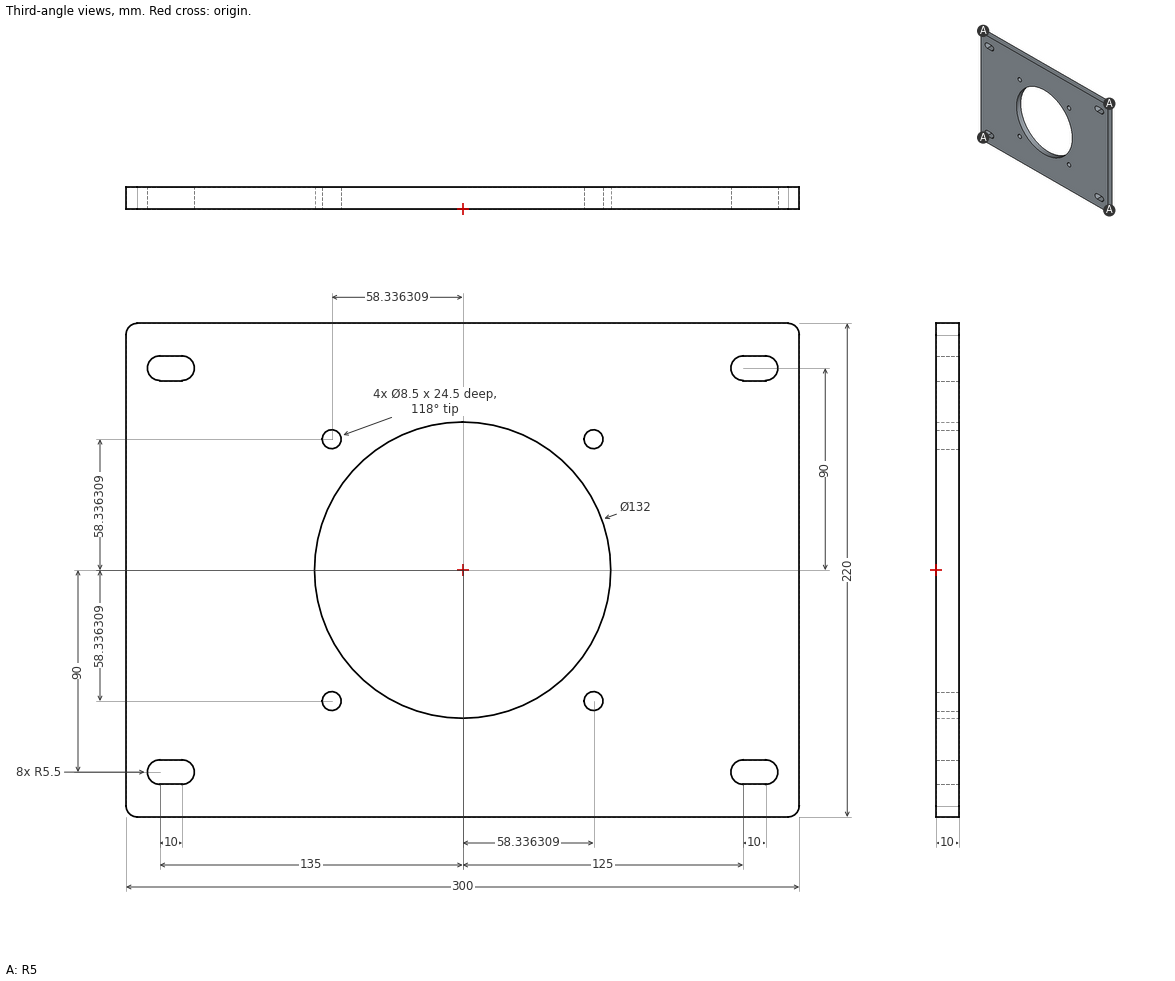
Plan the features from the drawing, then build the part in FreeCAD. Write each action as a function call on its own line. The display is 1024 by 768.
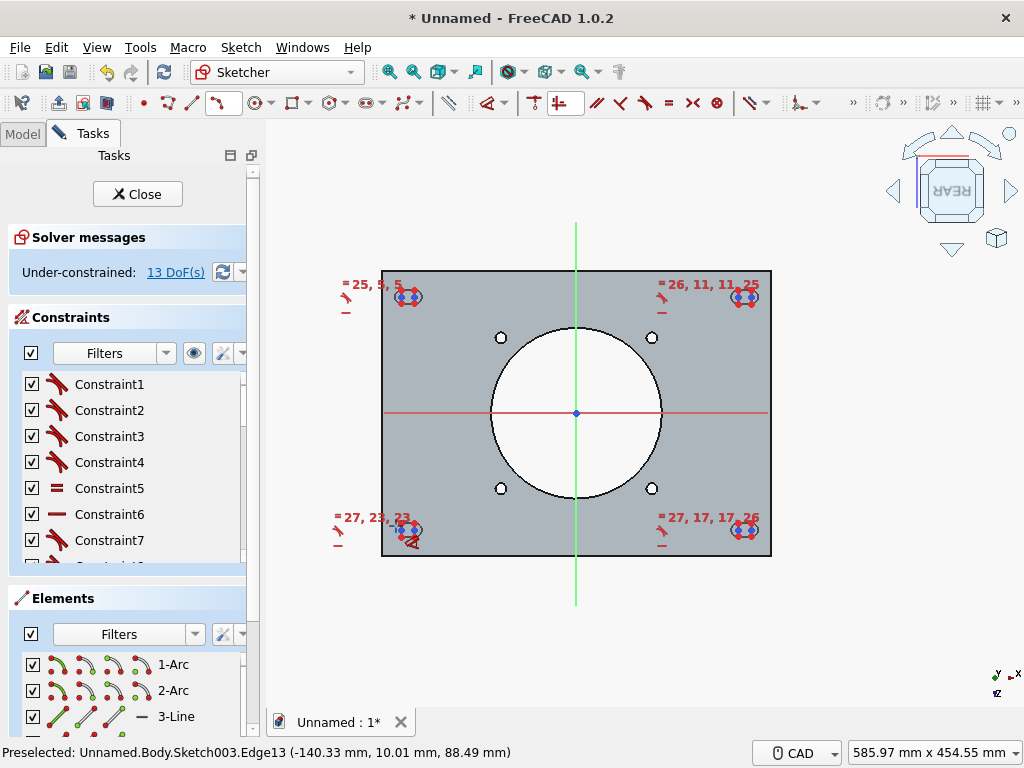
scroll(396, 293, up, 9)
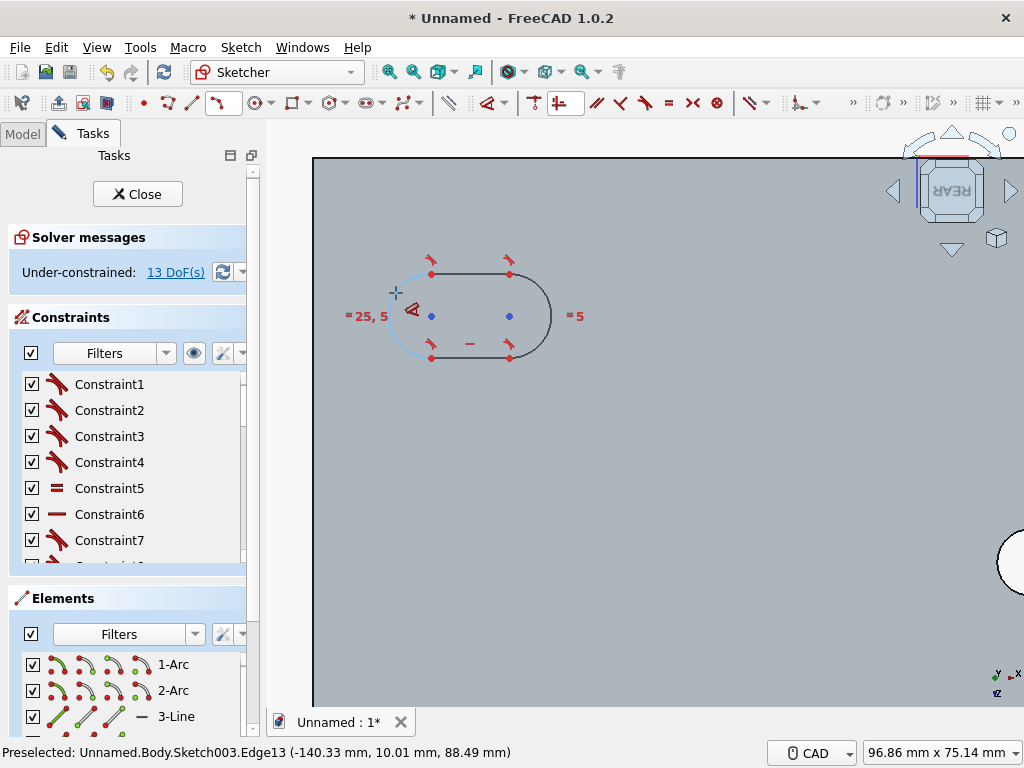
click(397, 291)
click(371, 272)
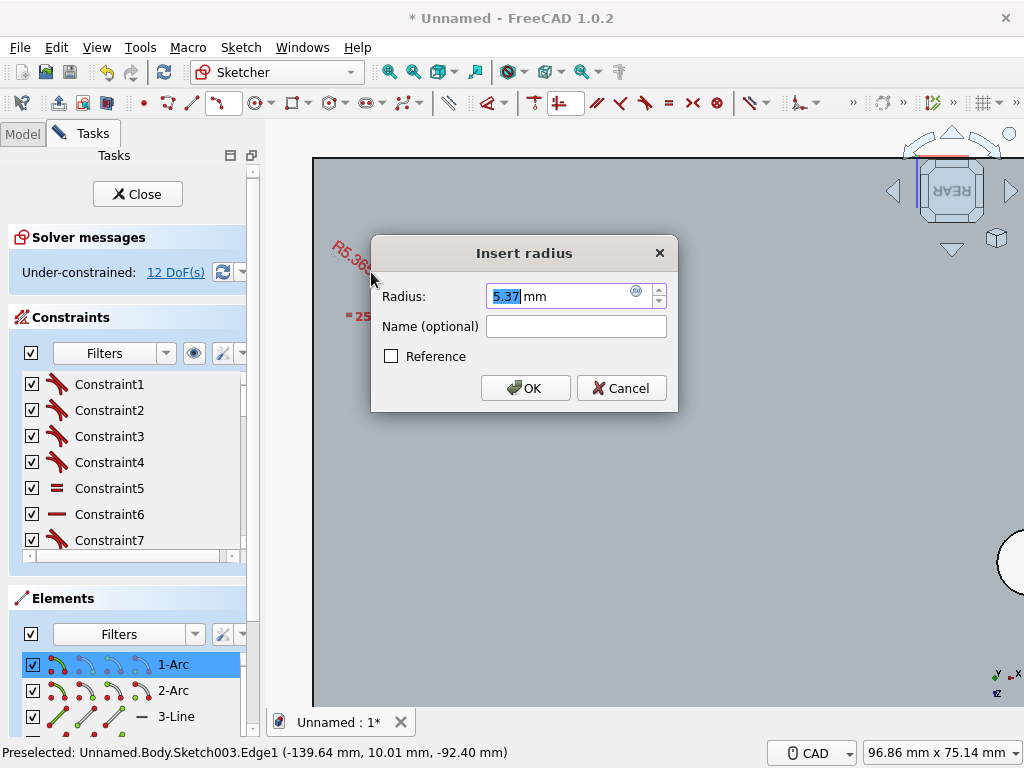
text(5.5)
key(Return)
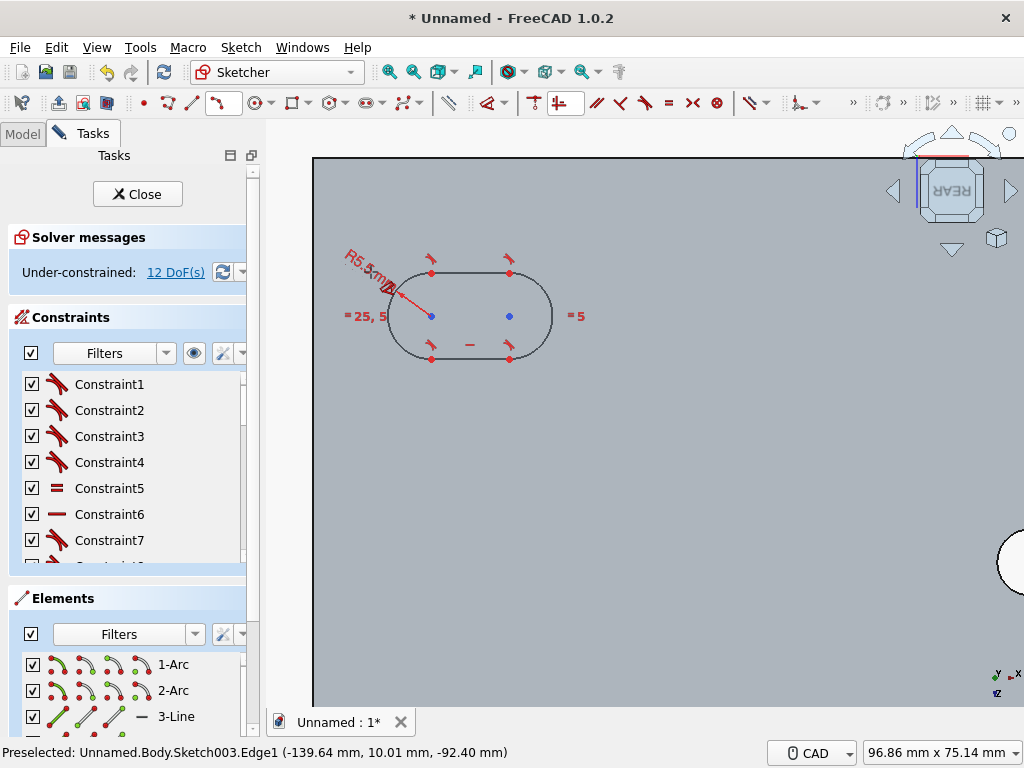
click(455, 273)
click(470, 239)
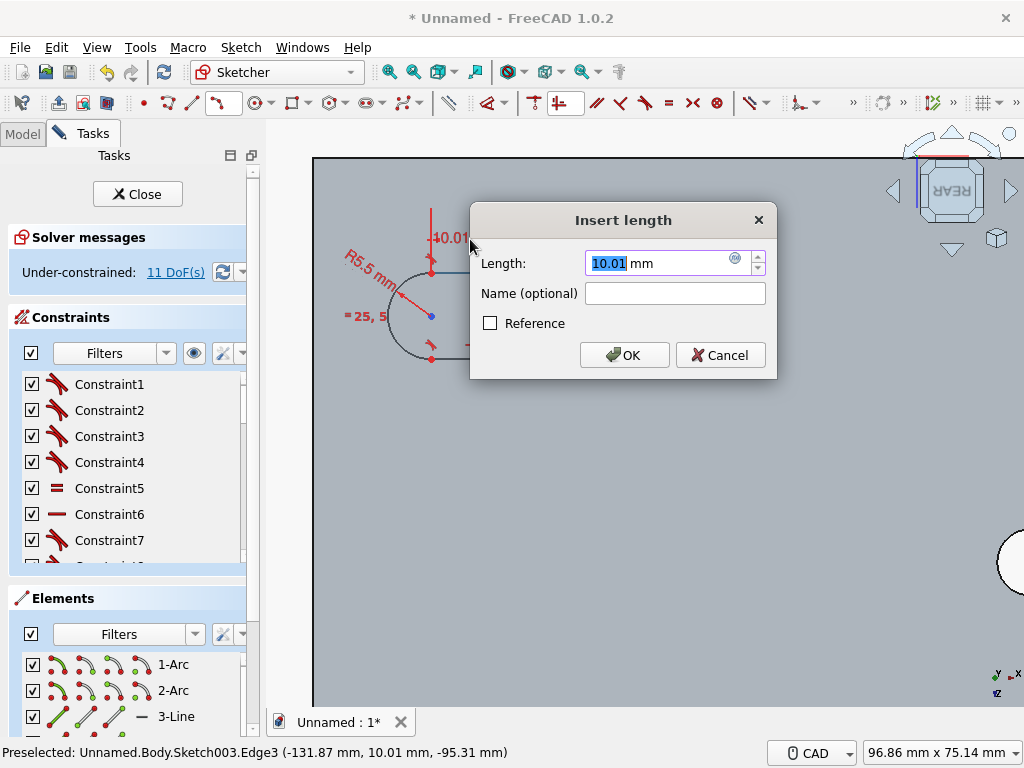
text(10)
key(Return)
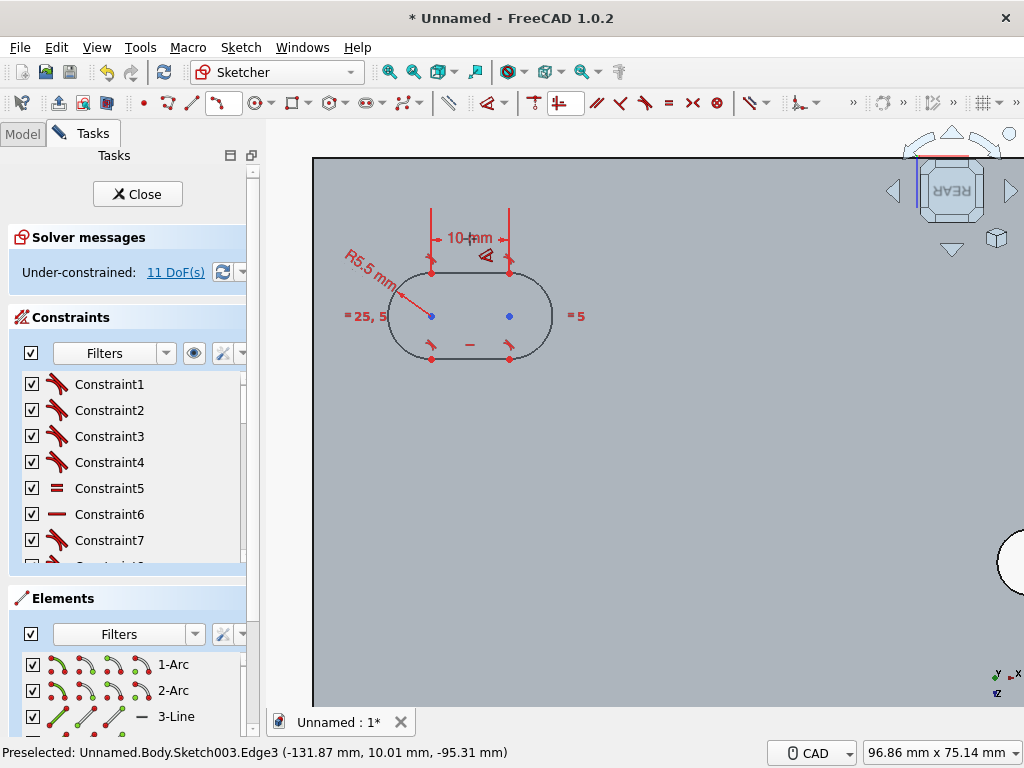
scroll(396, 293, down, 9)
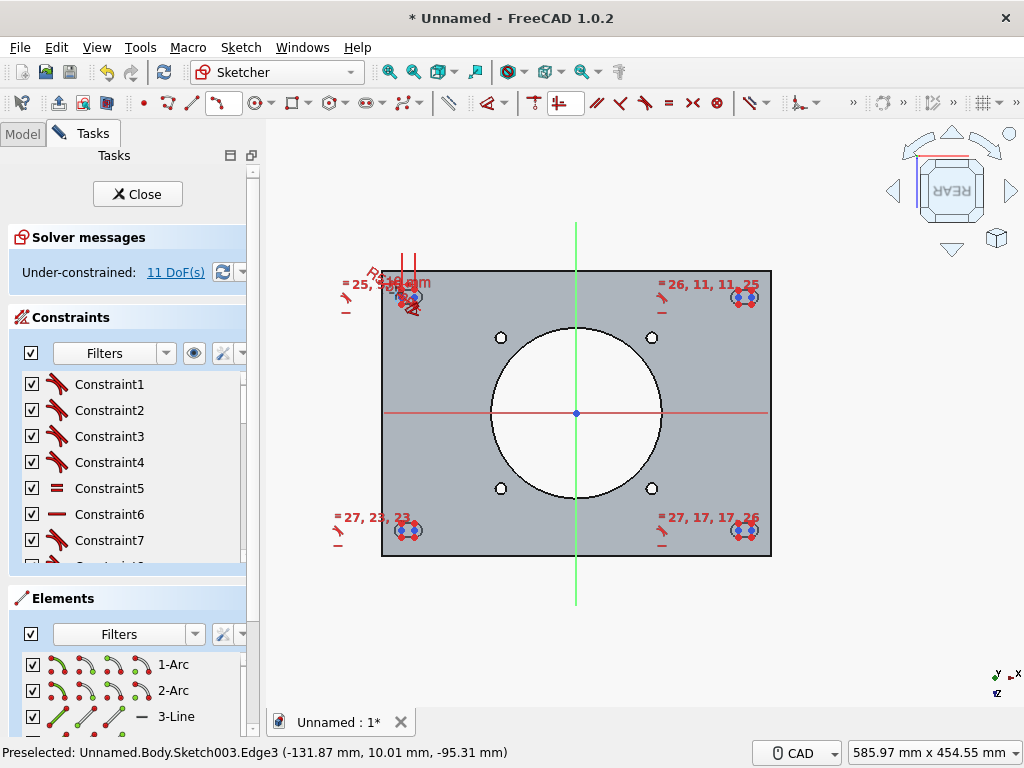
scroll(742, 290, up, 7)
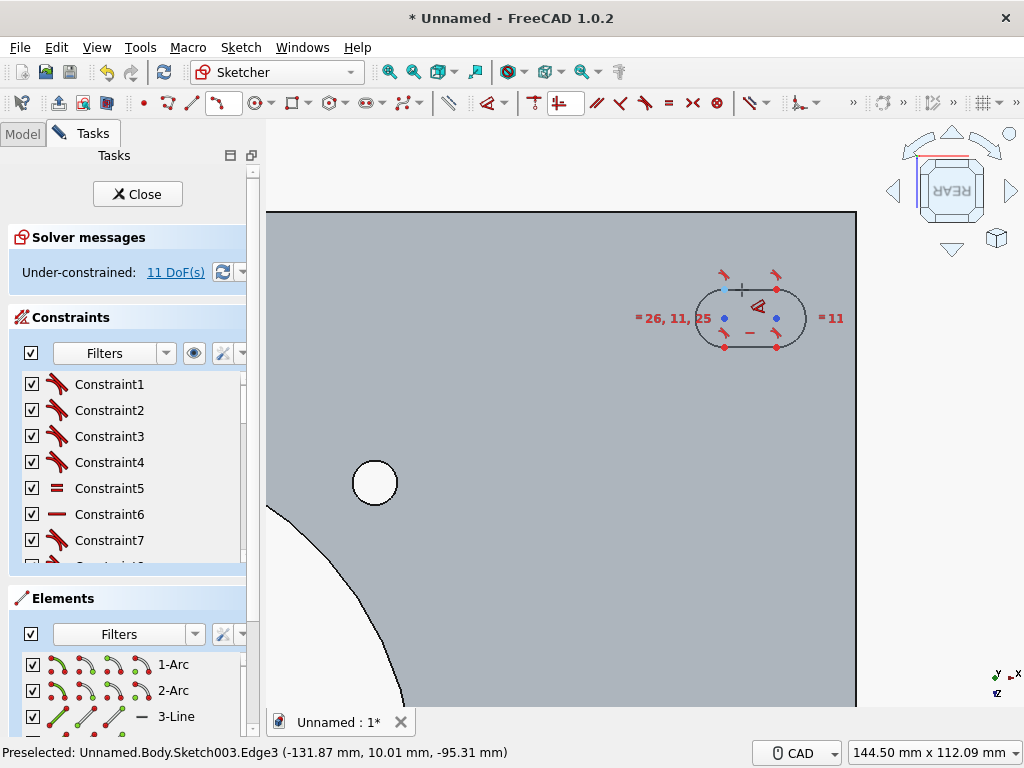
click(740, 290)
click(751, 256)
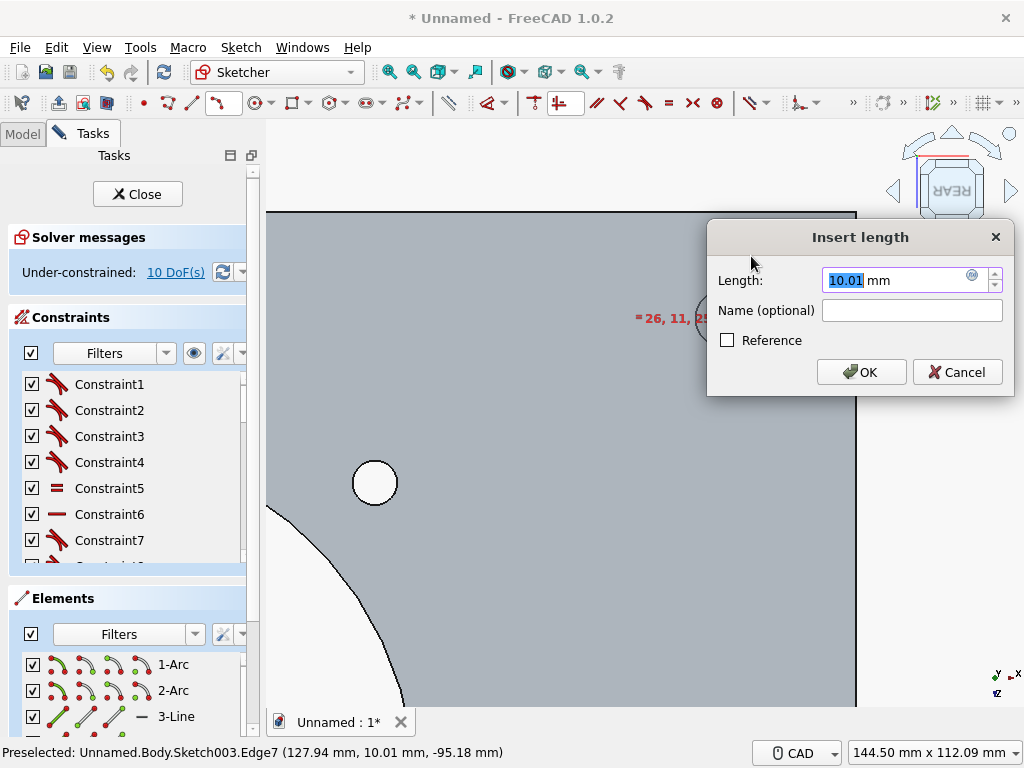
text(10)
key(Return)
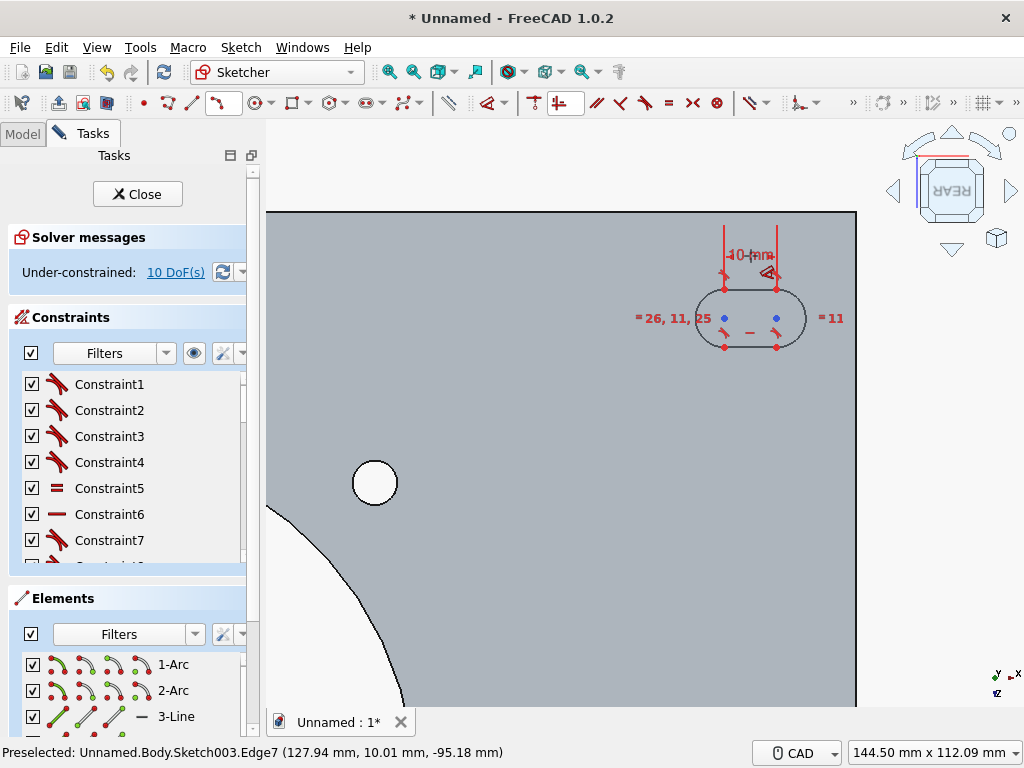
scroll(743, 290, down, 7)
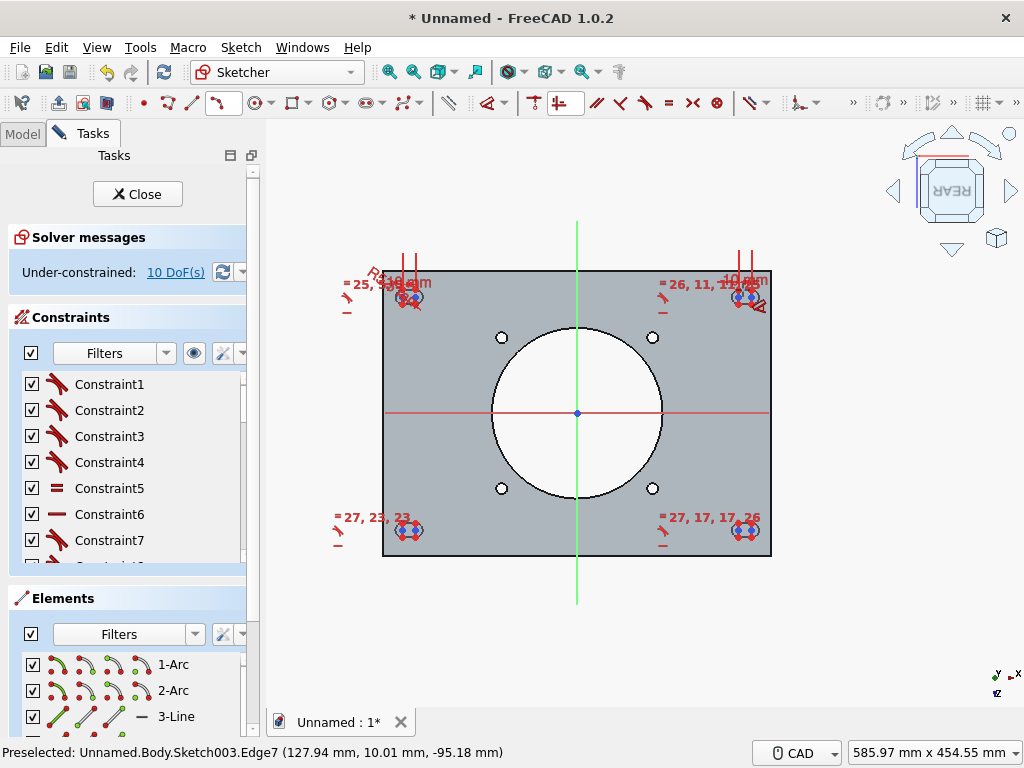
scroll(743, 523, up, 7)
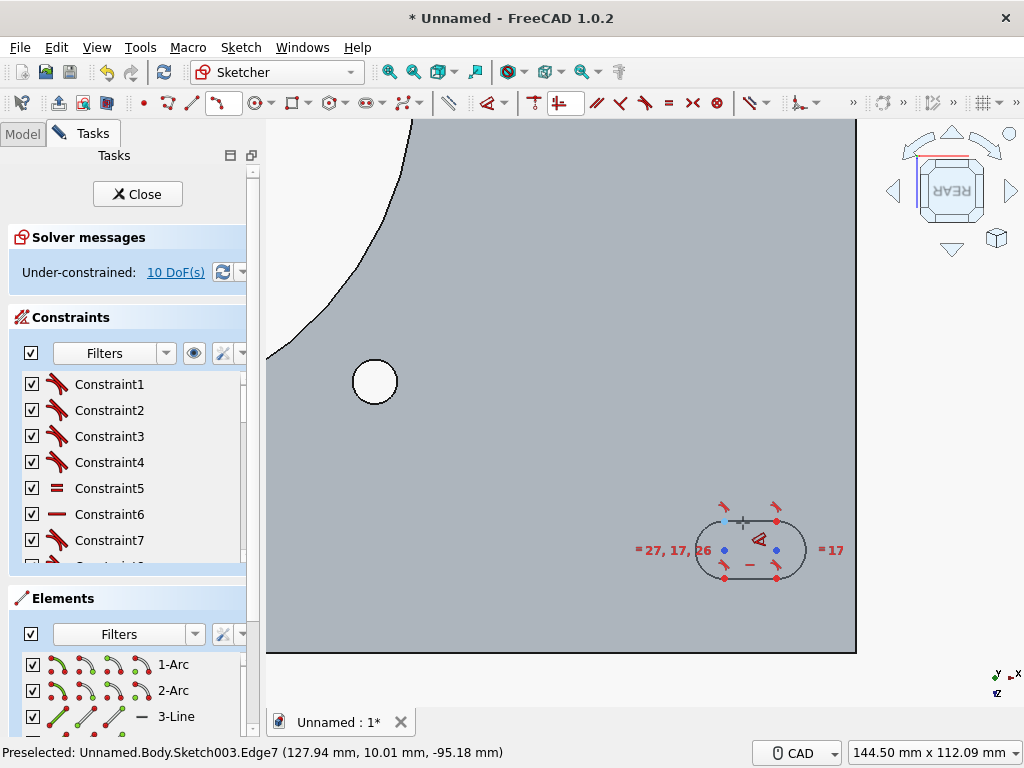
click(740, 521)
click(751, 555)